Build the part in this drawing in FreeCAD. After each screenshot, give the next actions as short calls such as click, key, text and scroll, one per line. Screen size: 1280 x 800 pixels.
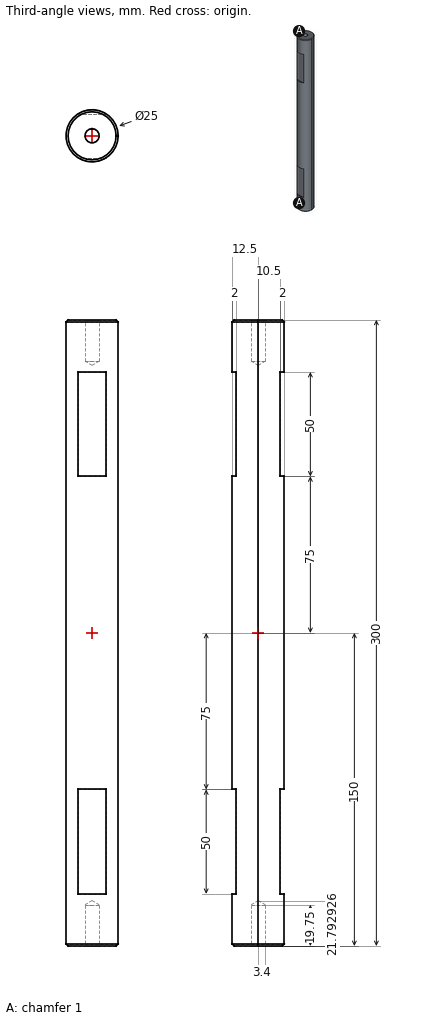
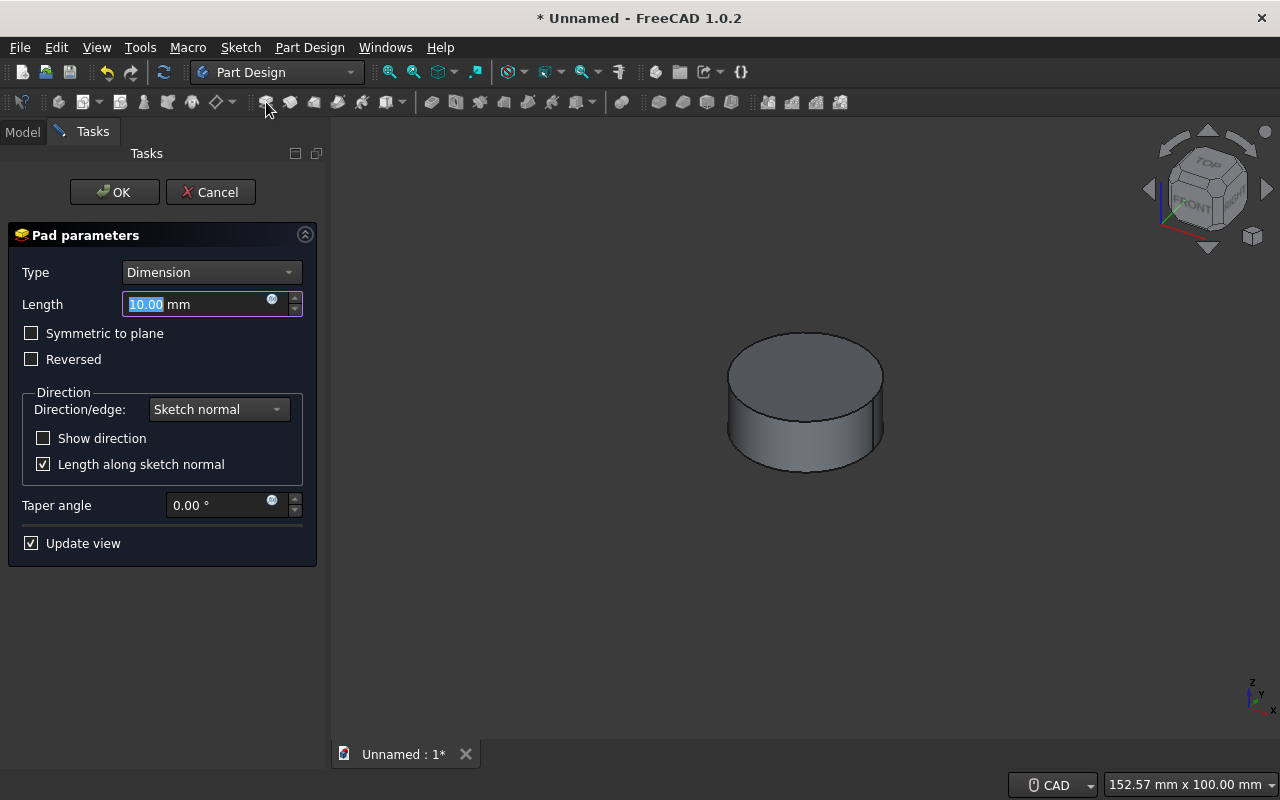
text(300)
key(Tab)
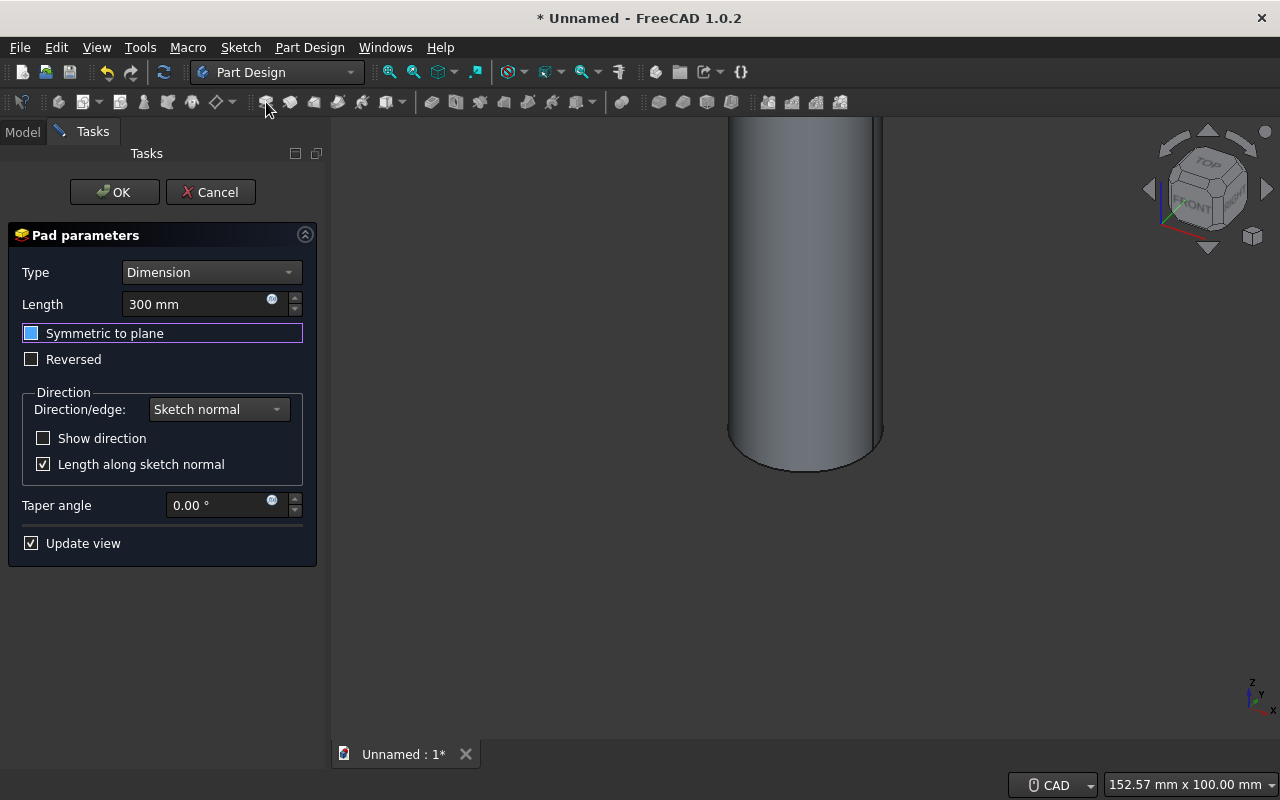
click(30, 333)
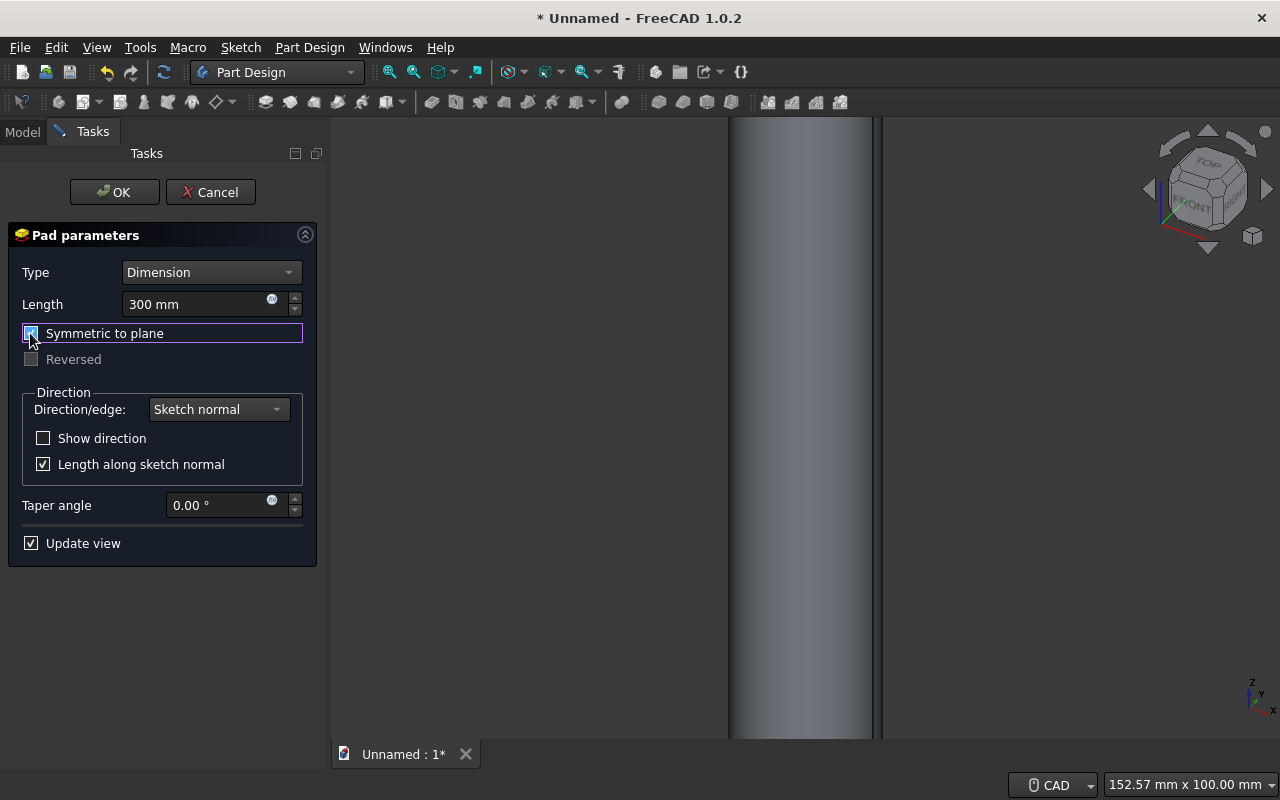
click(115, 192)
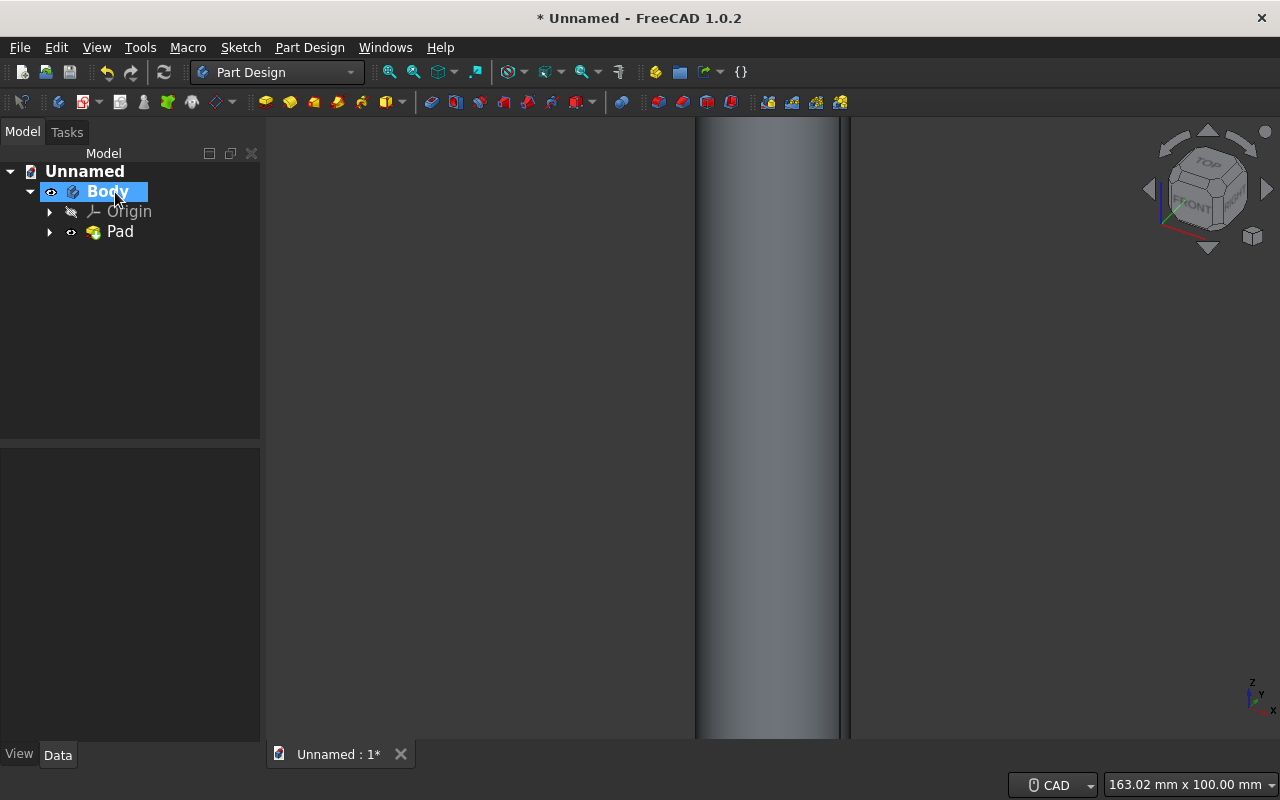
click(390, 72)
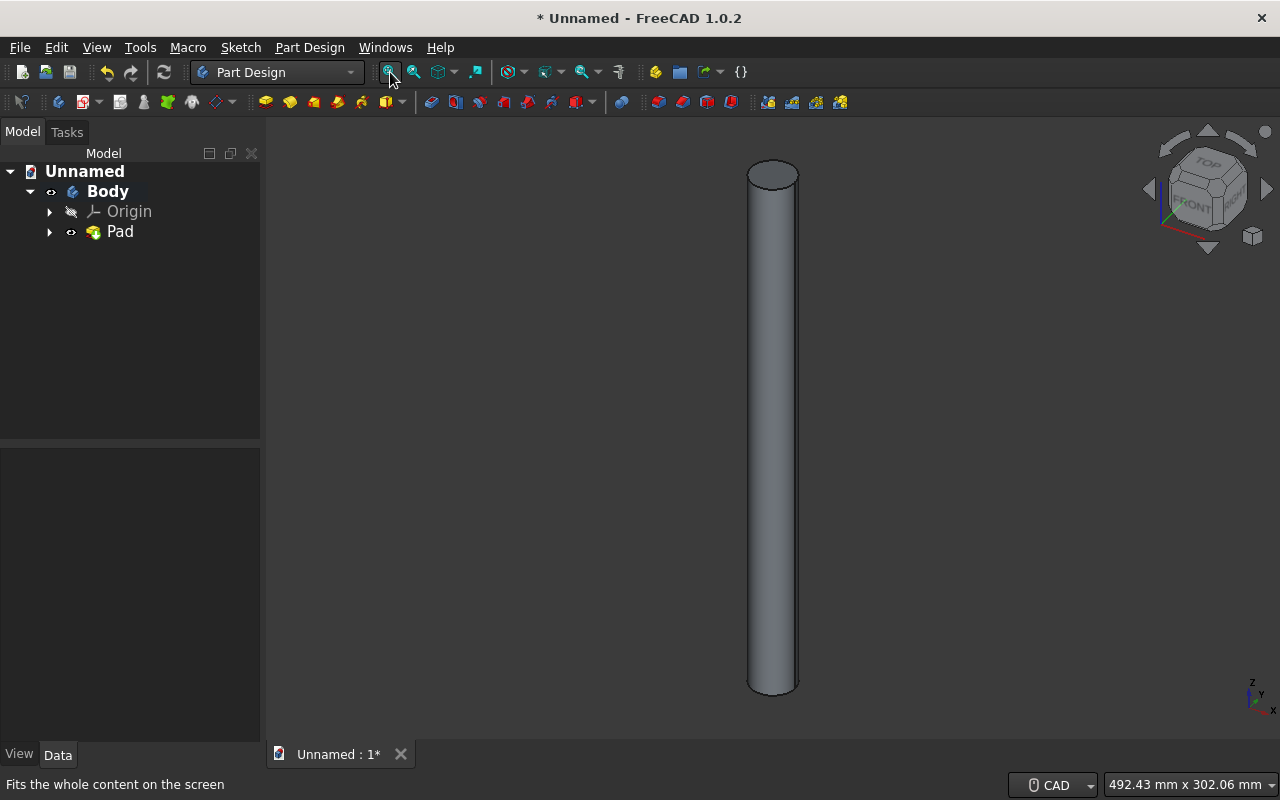
click(84, 102)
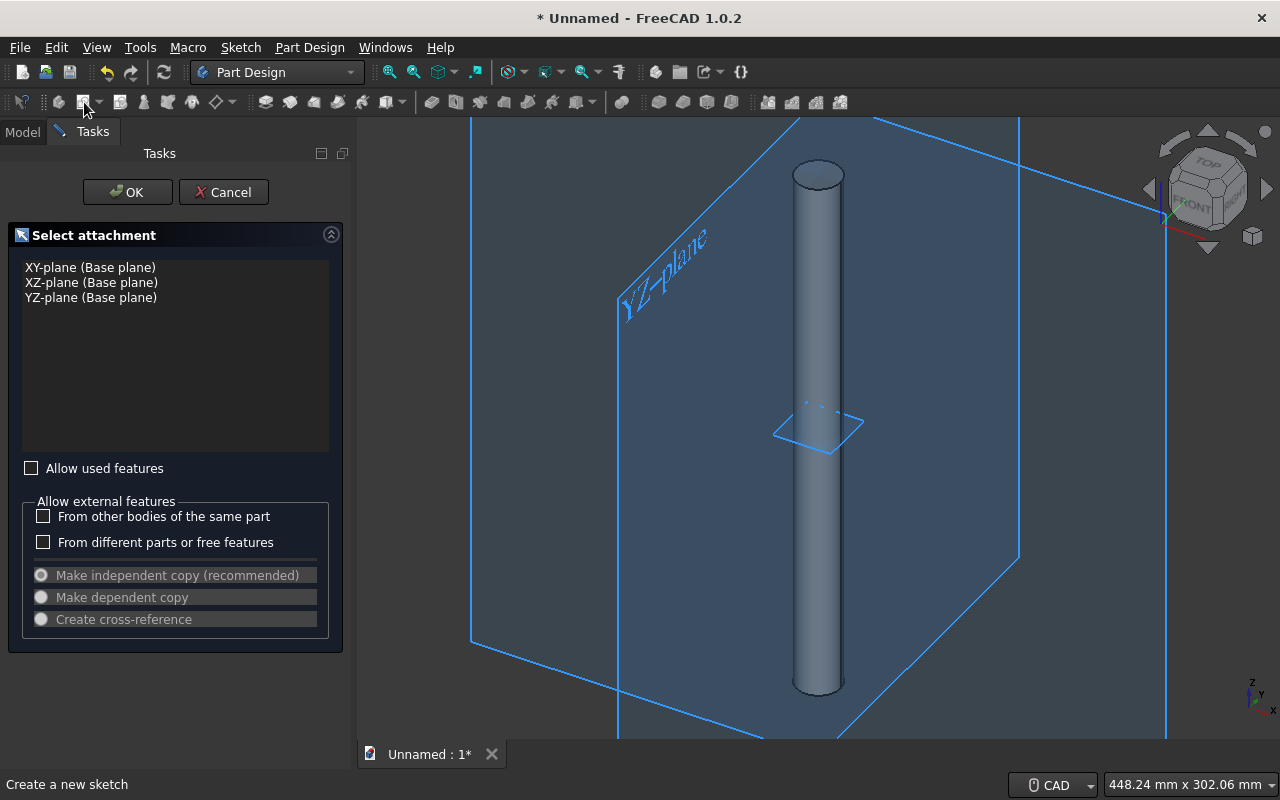
click(82, 298)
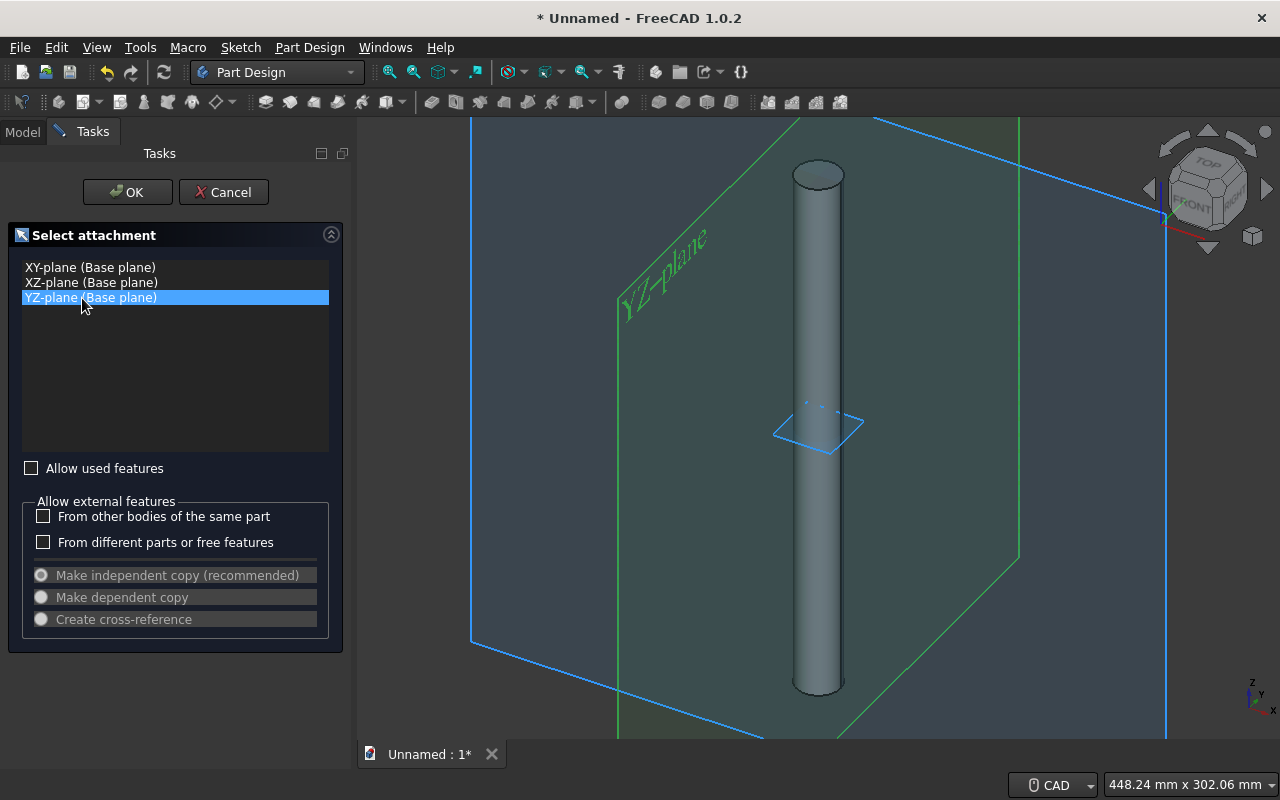
click(128, 192)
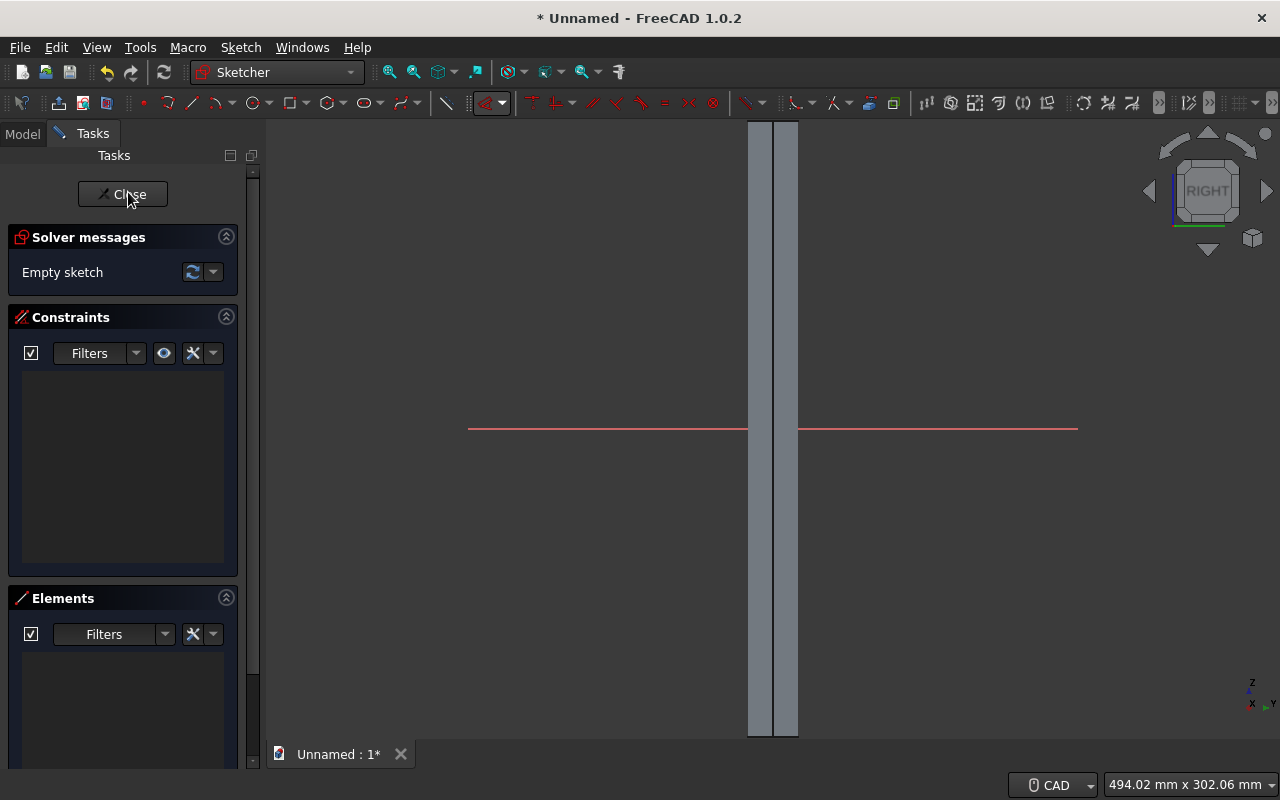
click(108, 104)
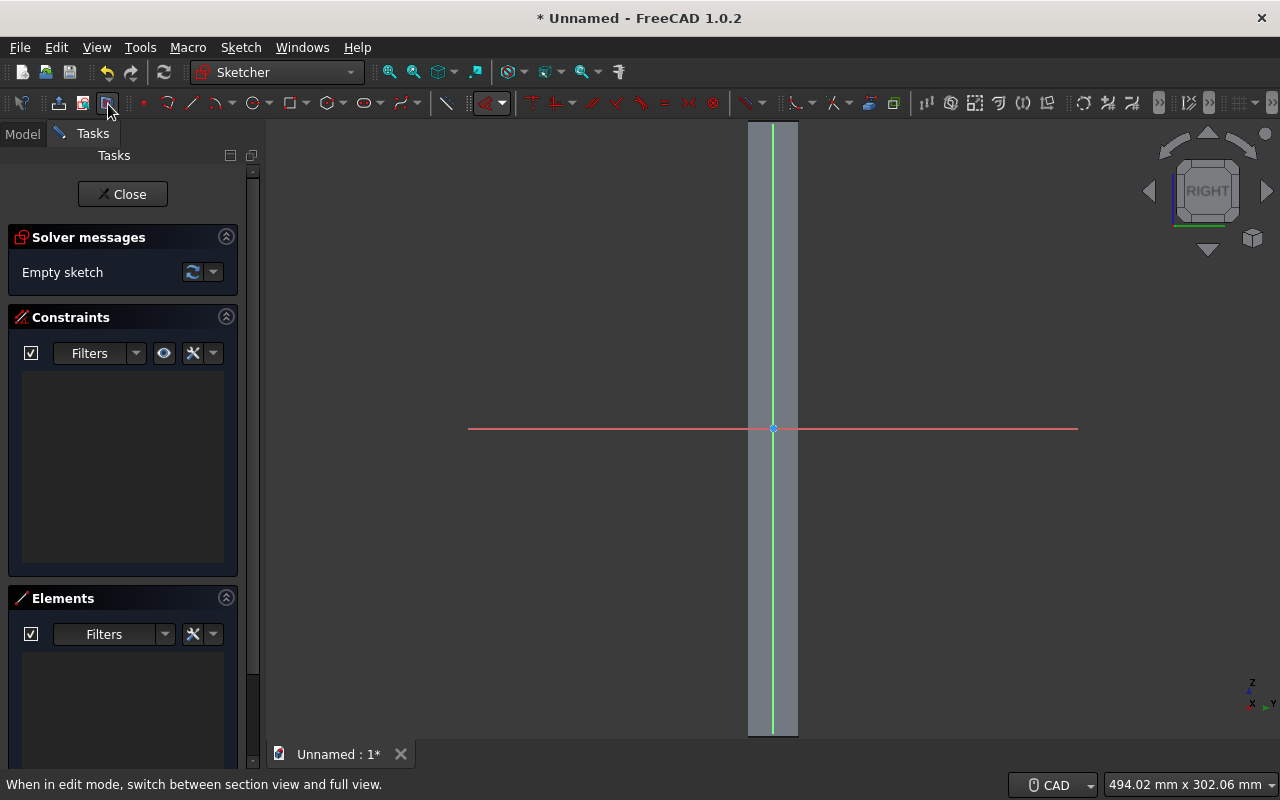
click(290, 104)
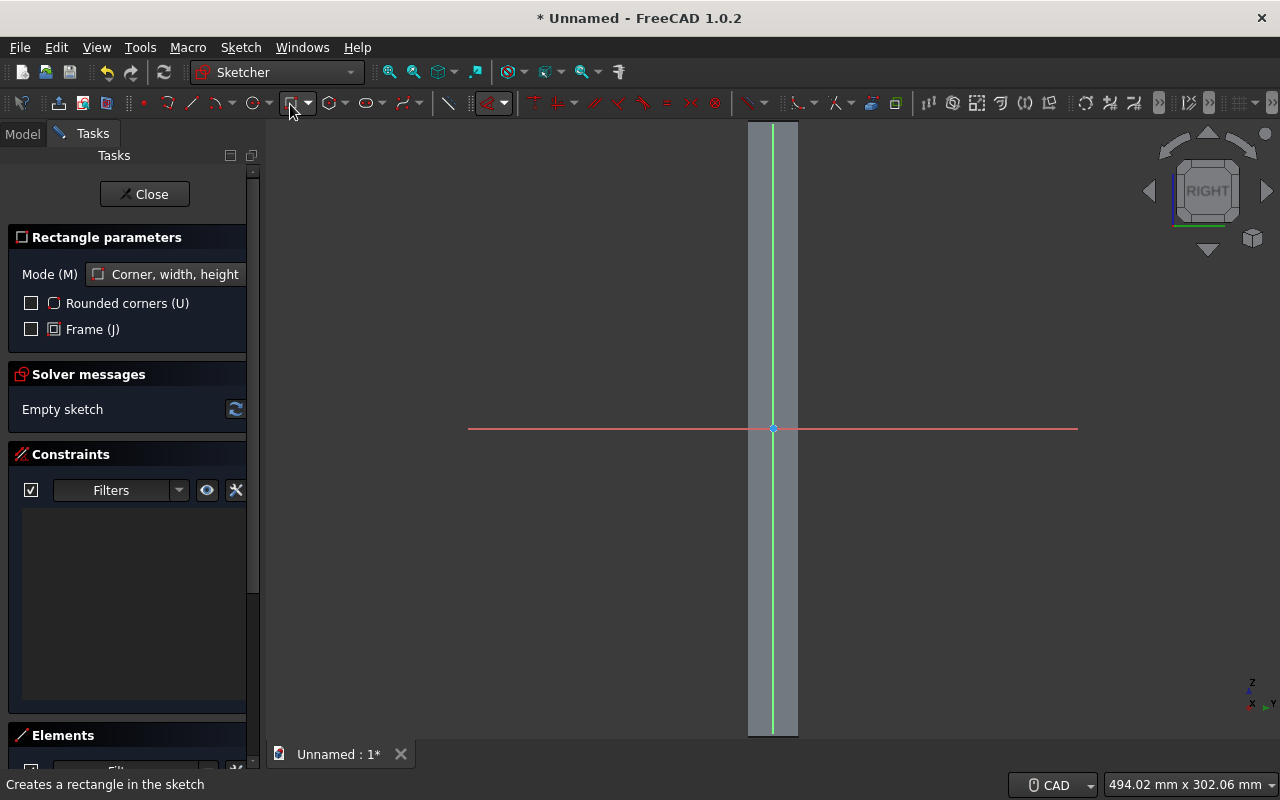
scroll(795, 172, up, 7)